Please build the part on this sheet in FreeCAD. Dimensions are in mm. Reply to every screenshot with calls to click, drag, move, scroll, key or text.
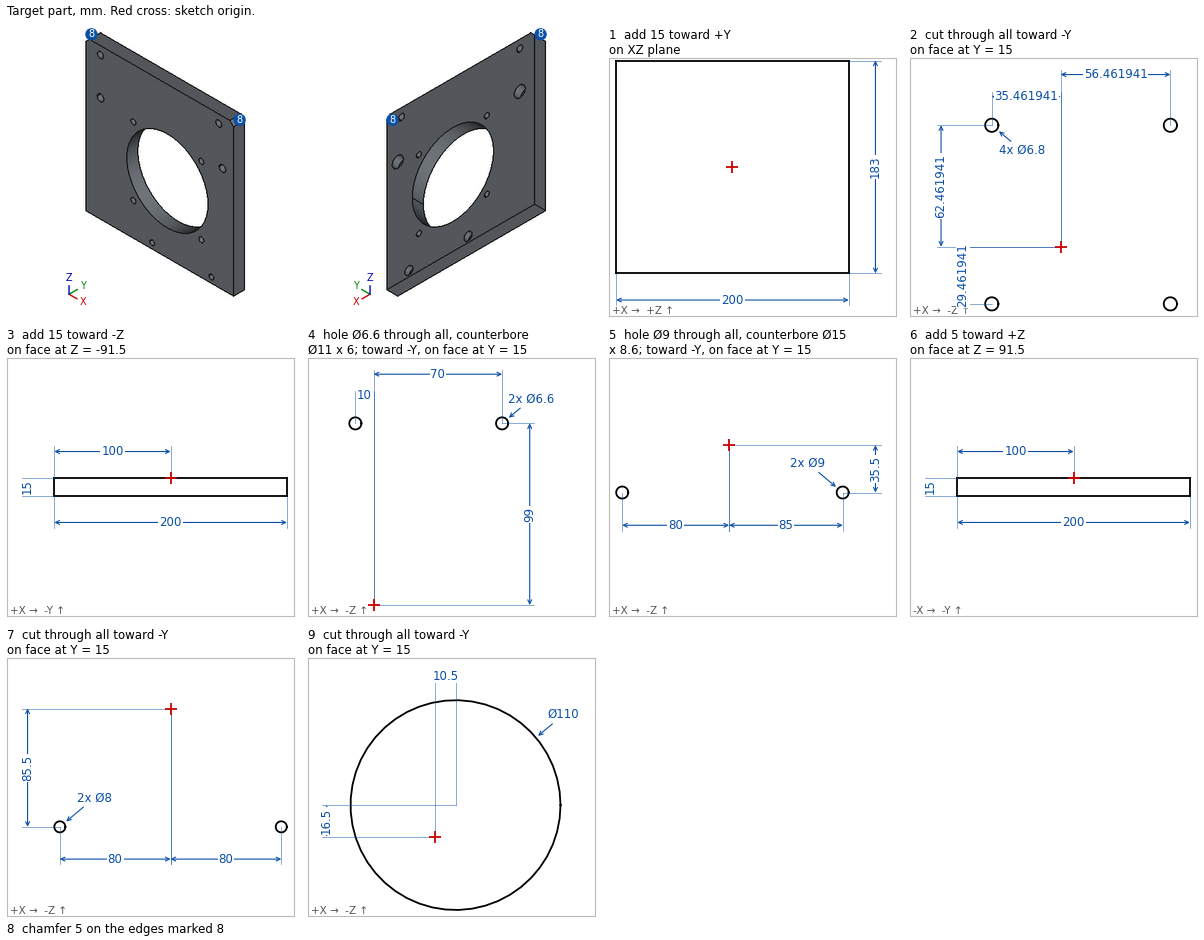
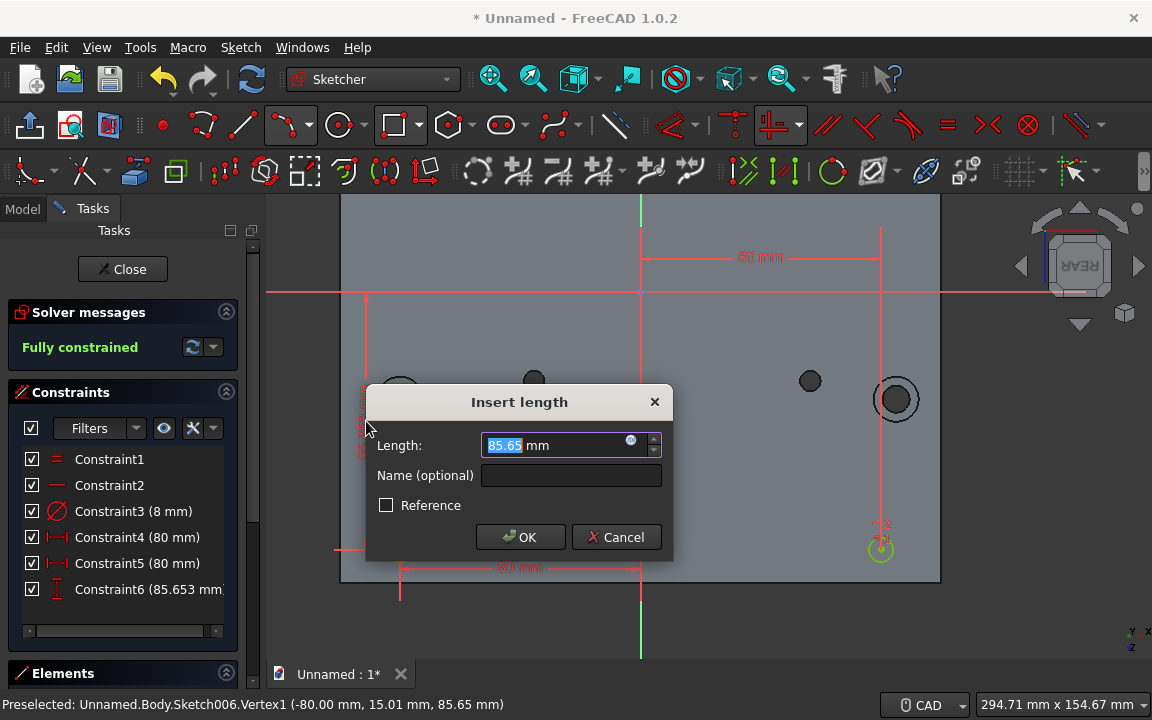
text(85.5)
key(Return)
key(Escape)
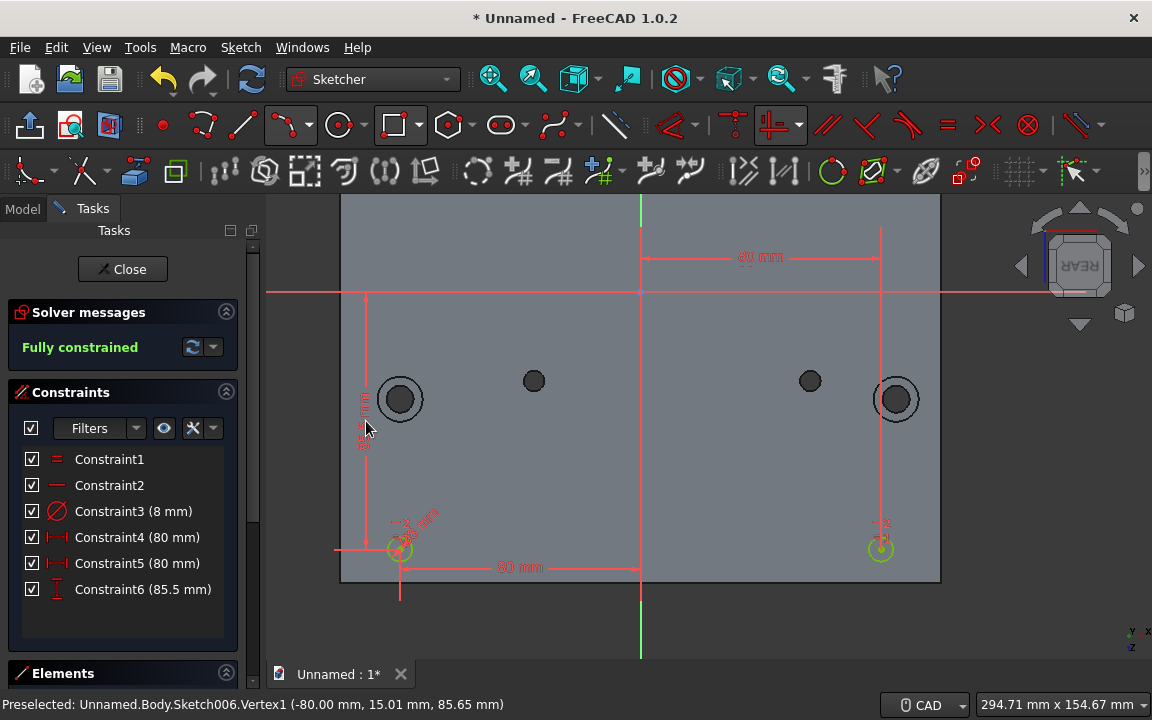
click(123, 269)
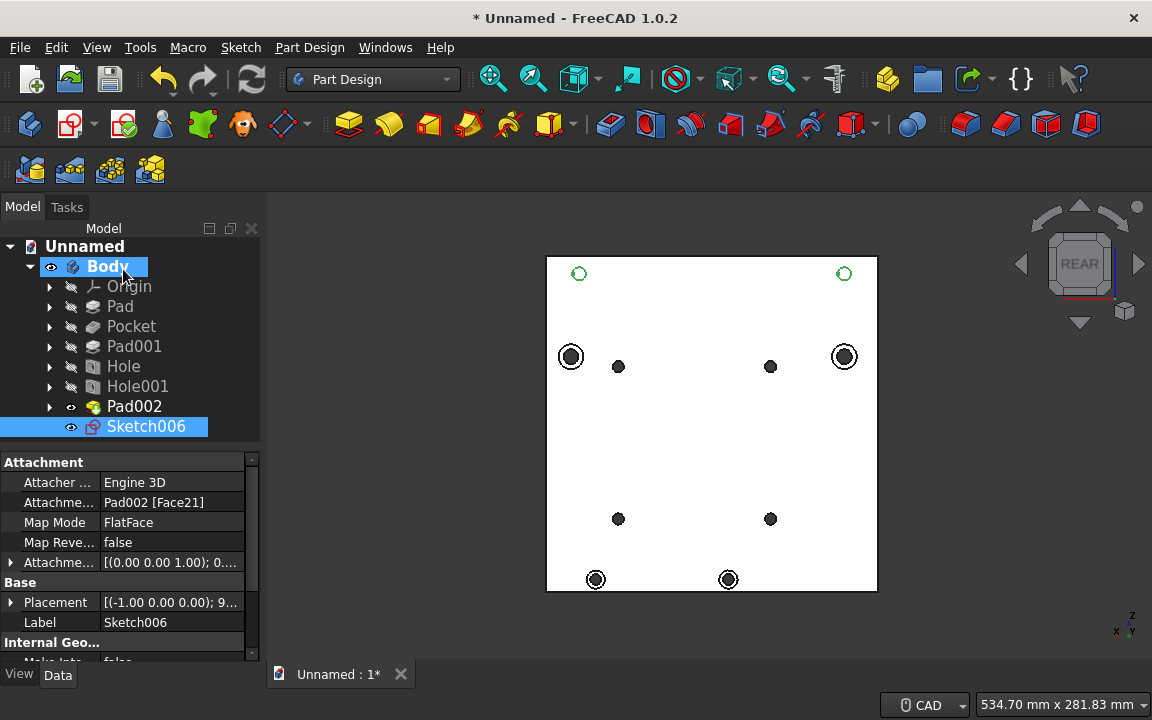
click(612, 124)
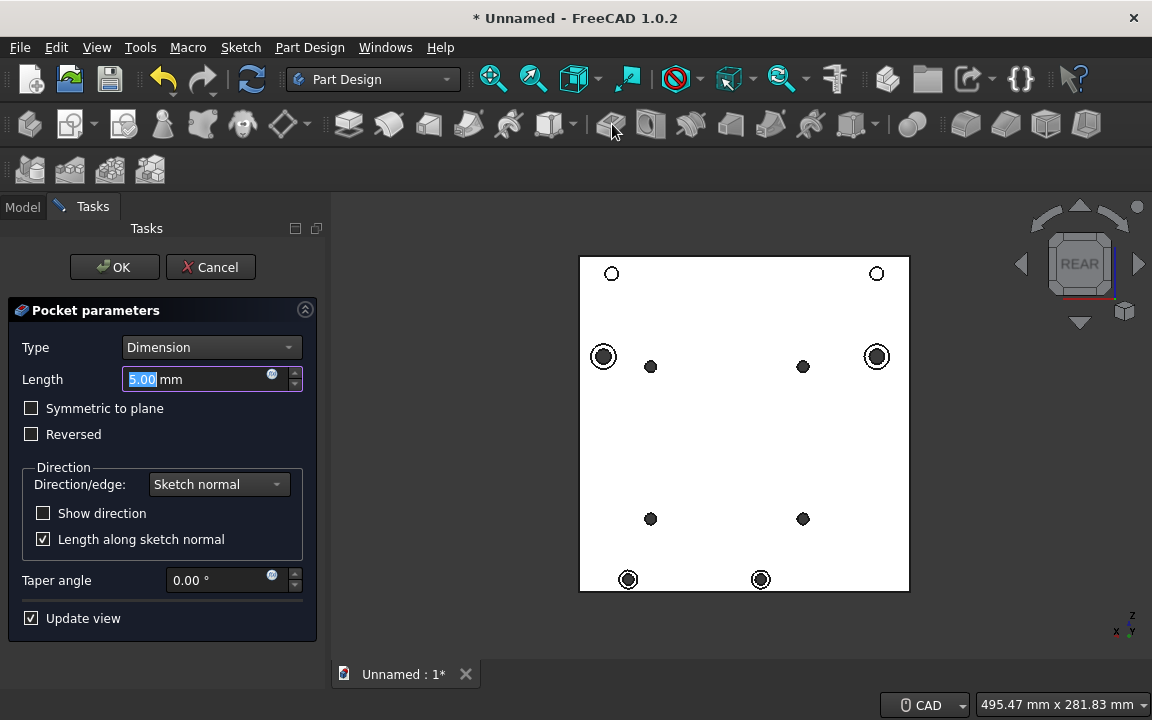
click(212, 348)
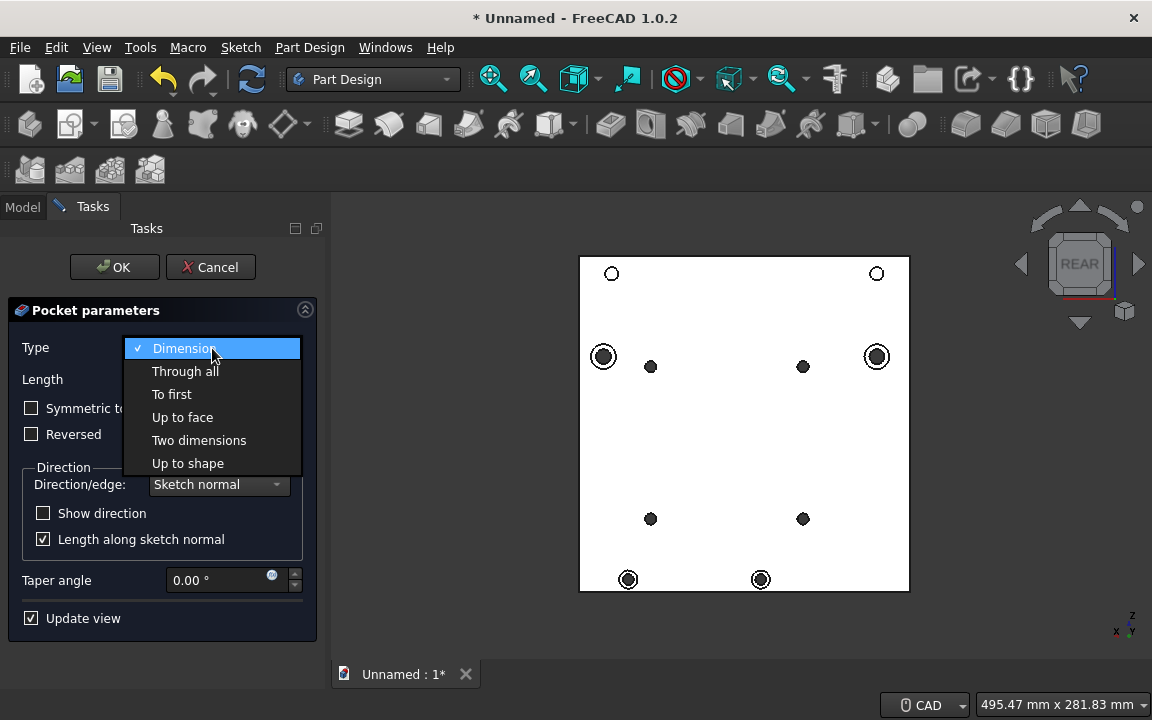
click(212, 372)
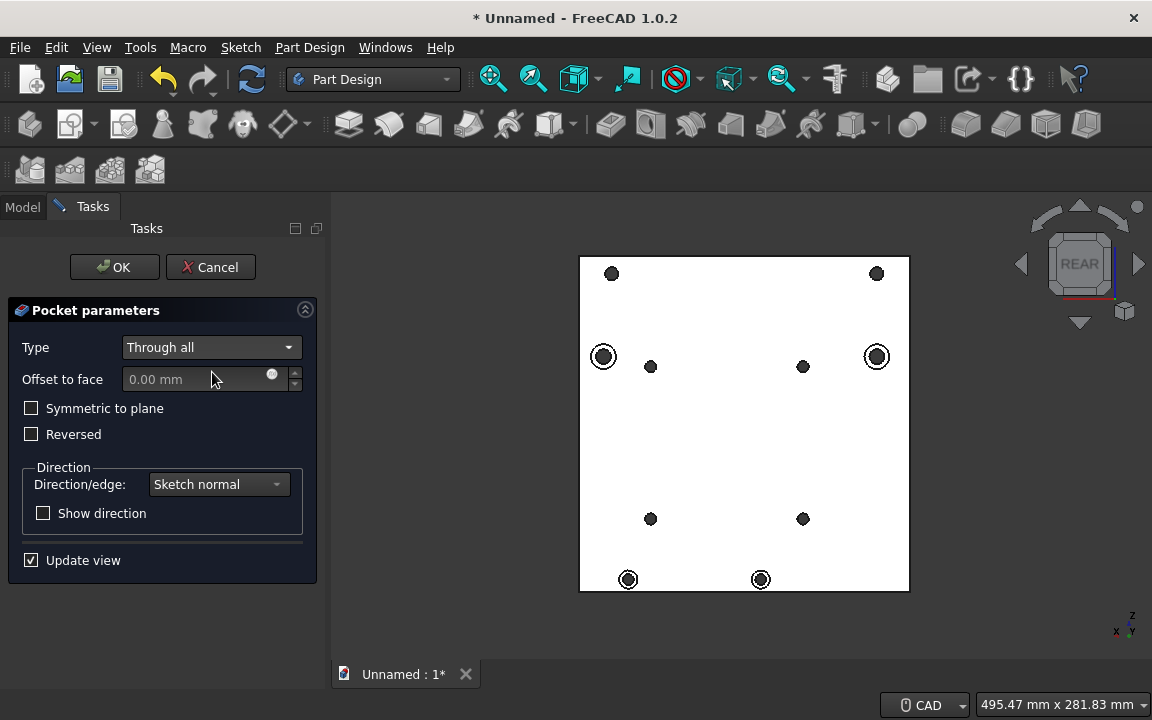
click(115, 267)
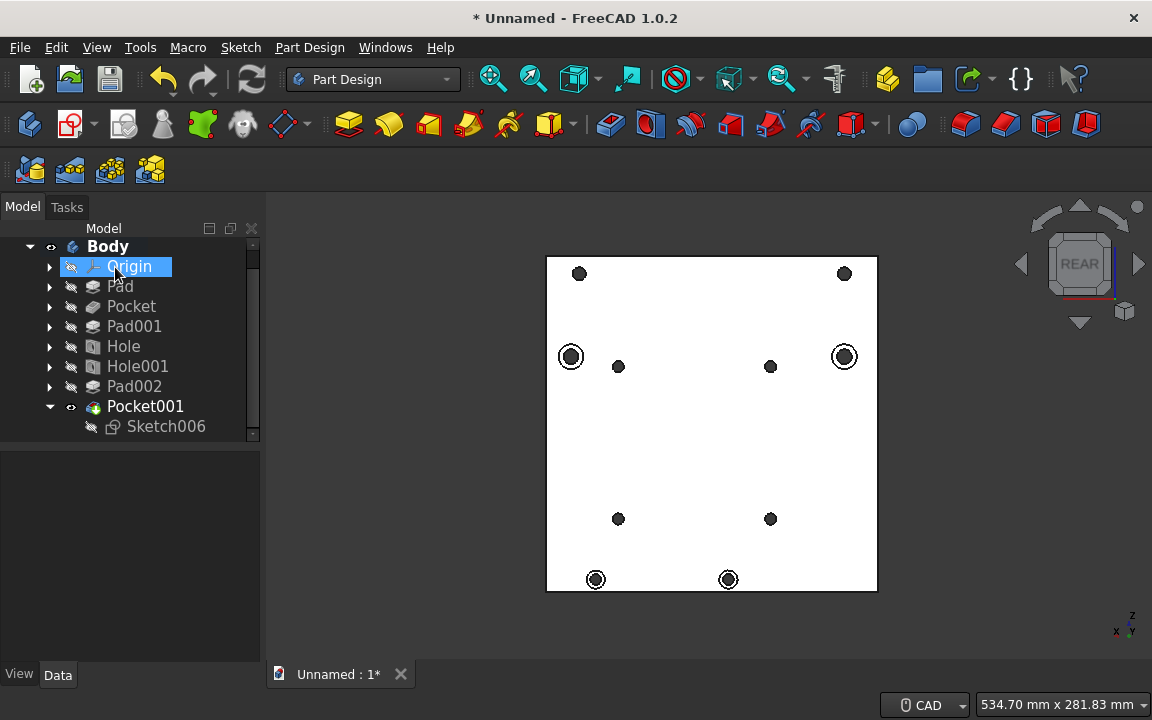
key(0)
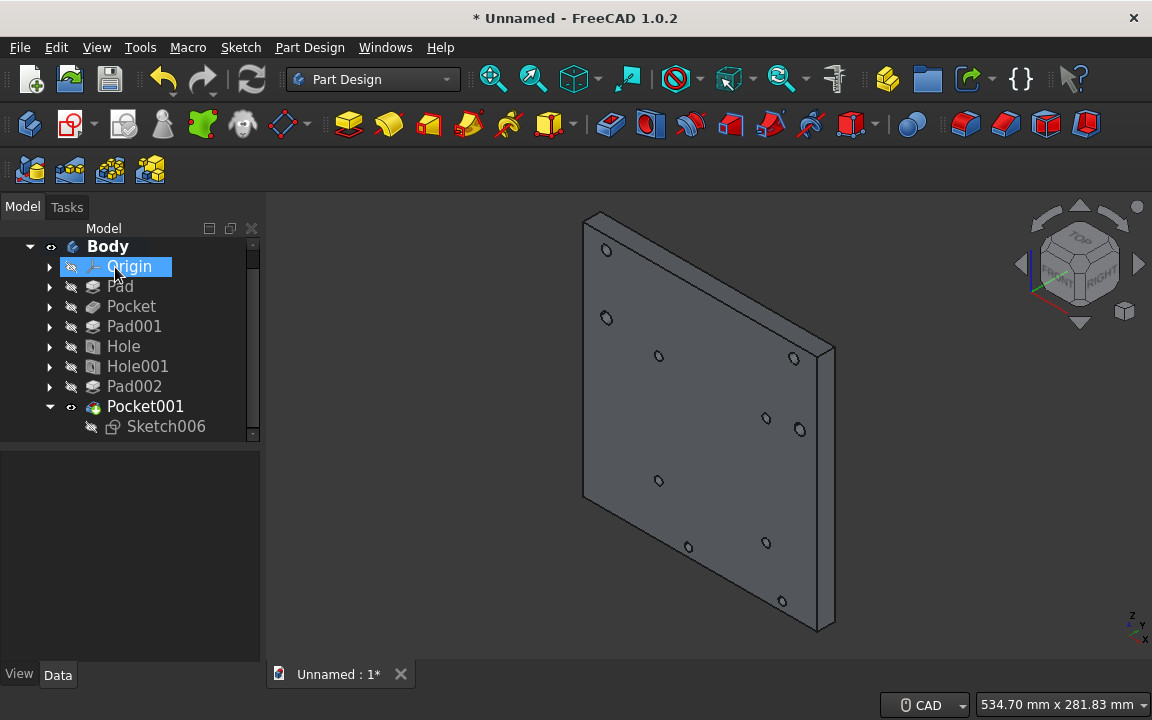
click(826, 351)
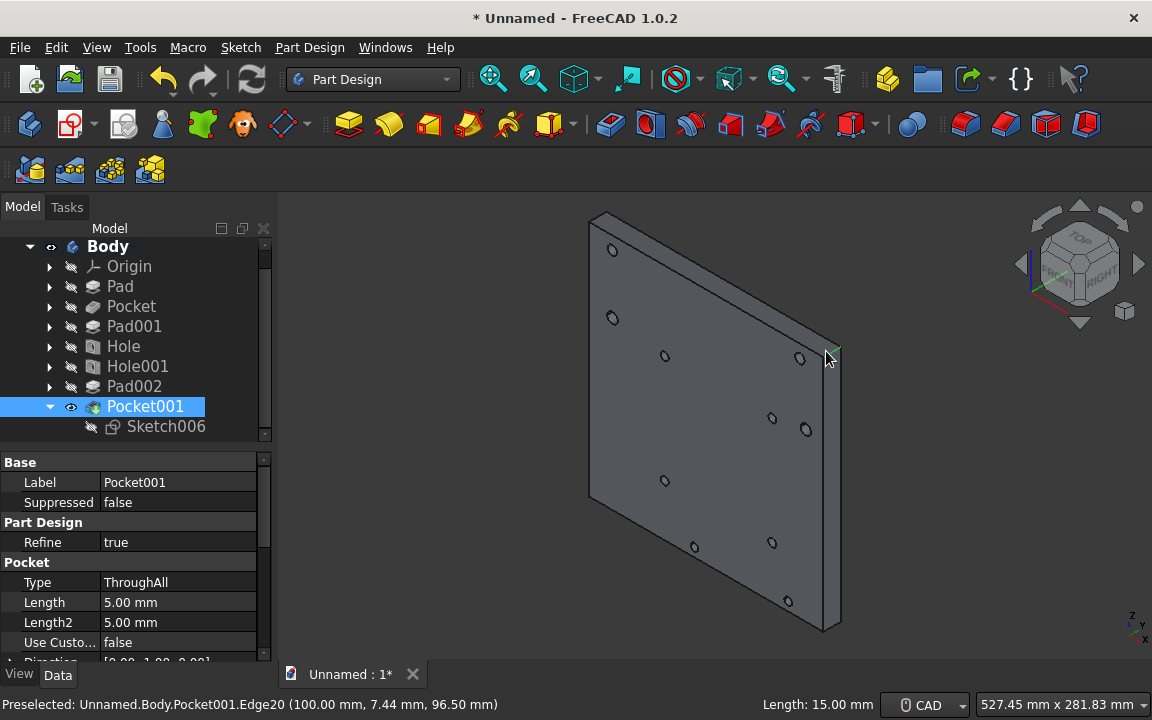
key(2)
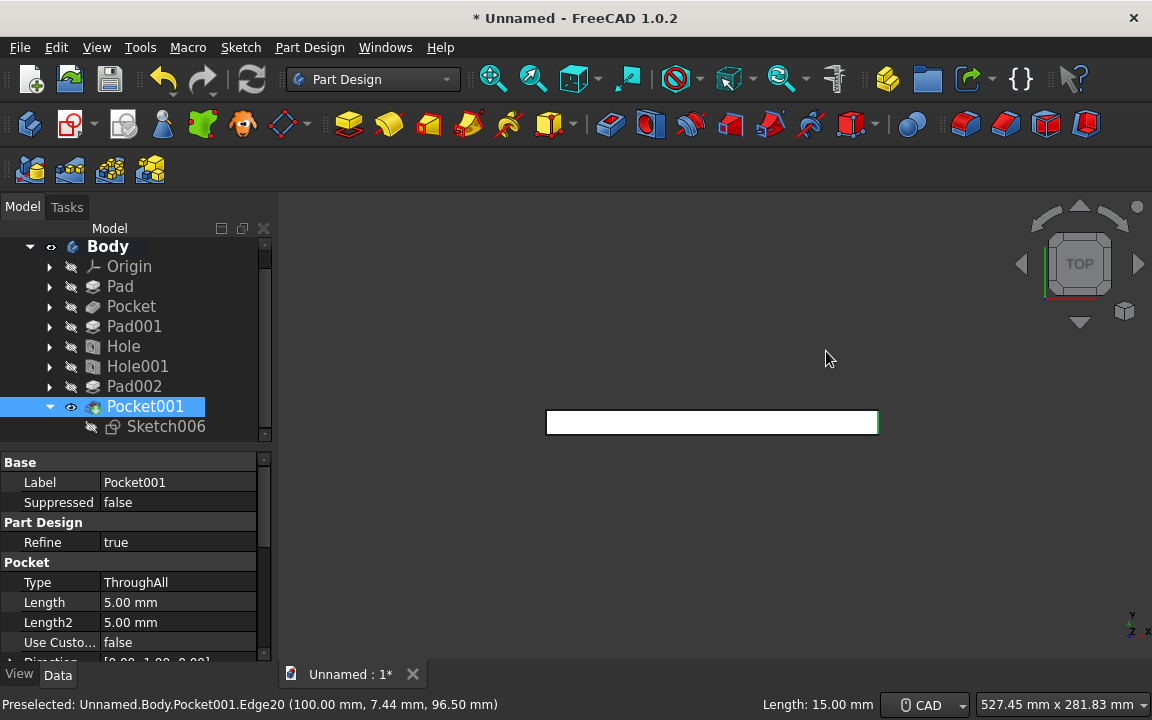
click(494, 80)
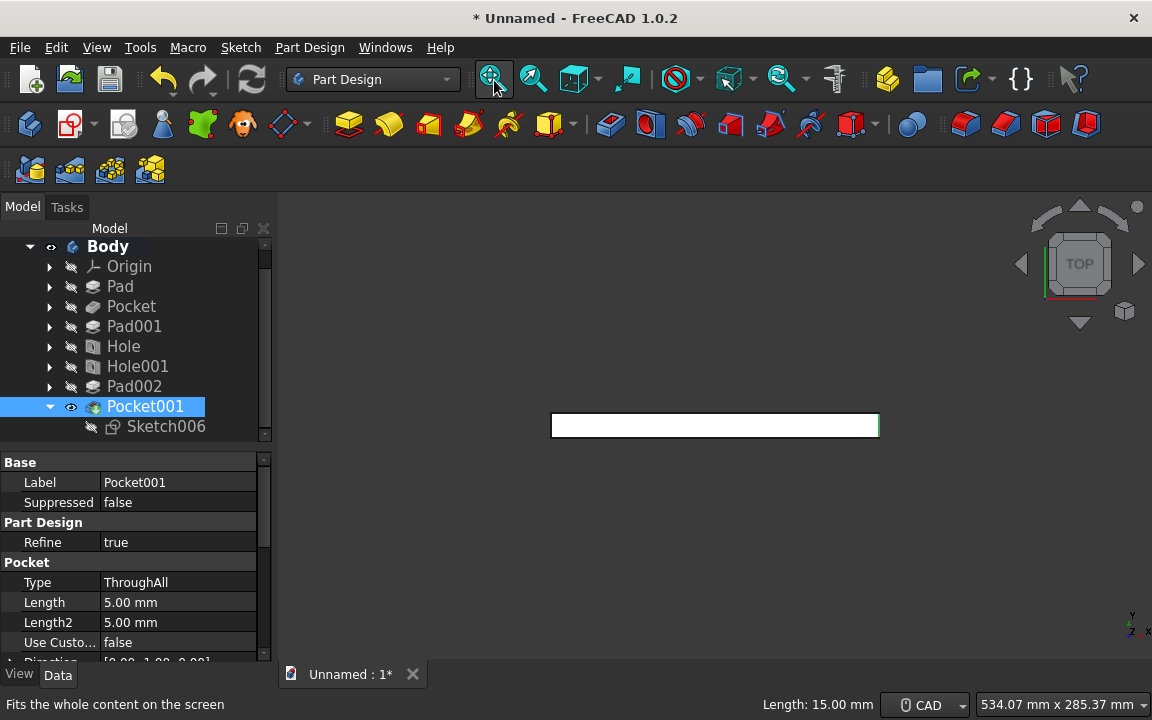
click(551, 424, ctrl)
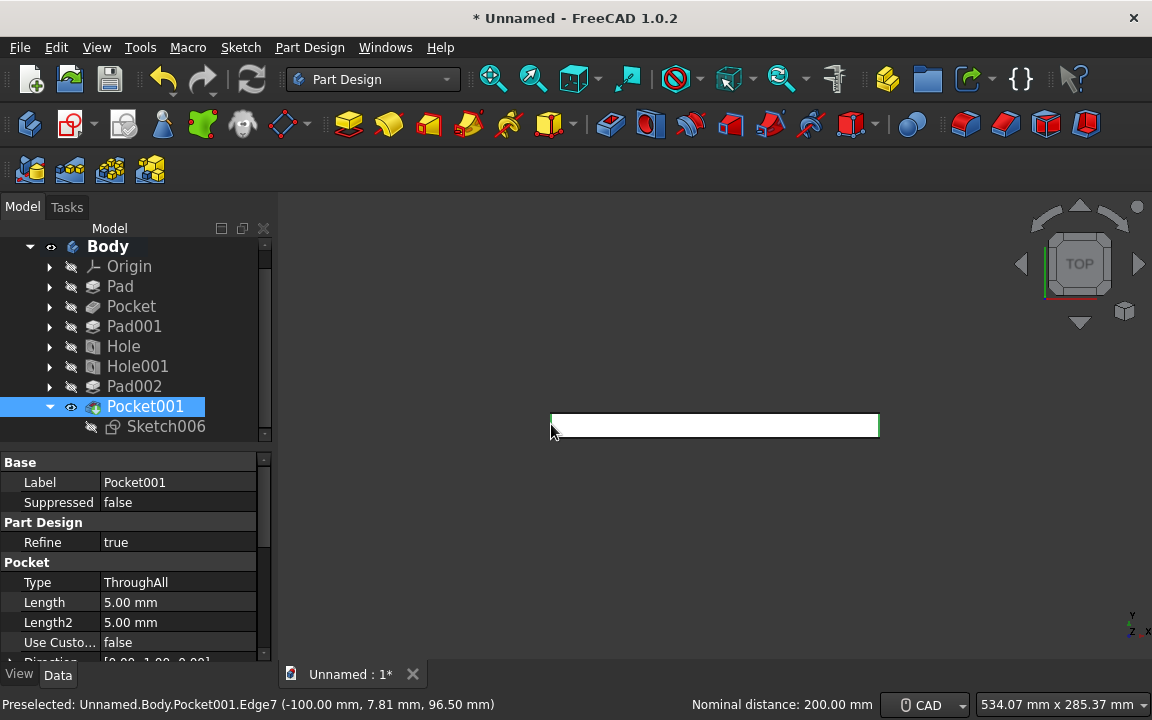
click(1006, 124)